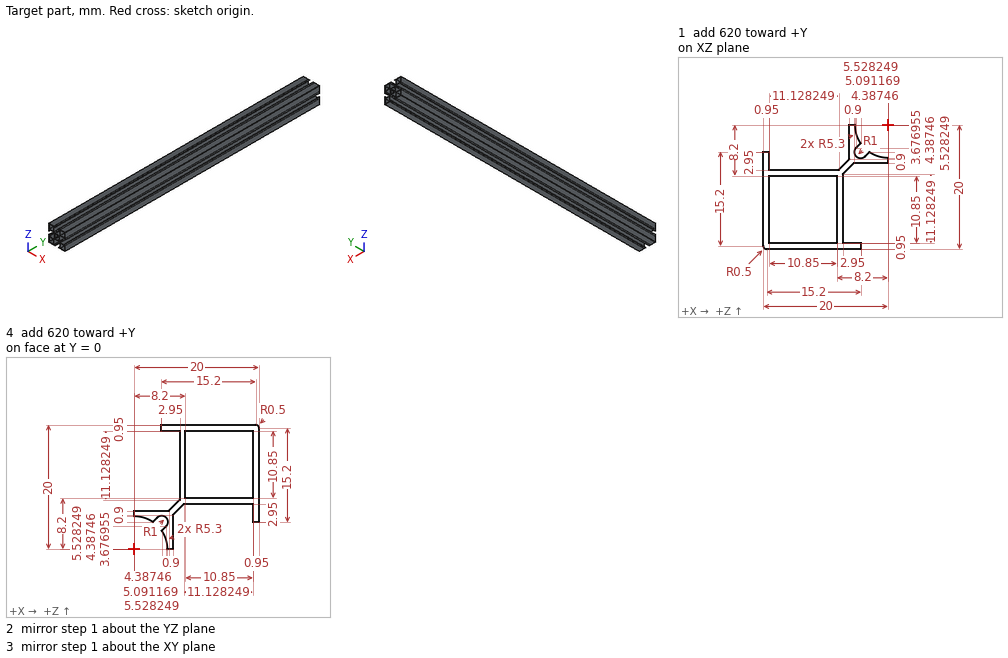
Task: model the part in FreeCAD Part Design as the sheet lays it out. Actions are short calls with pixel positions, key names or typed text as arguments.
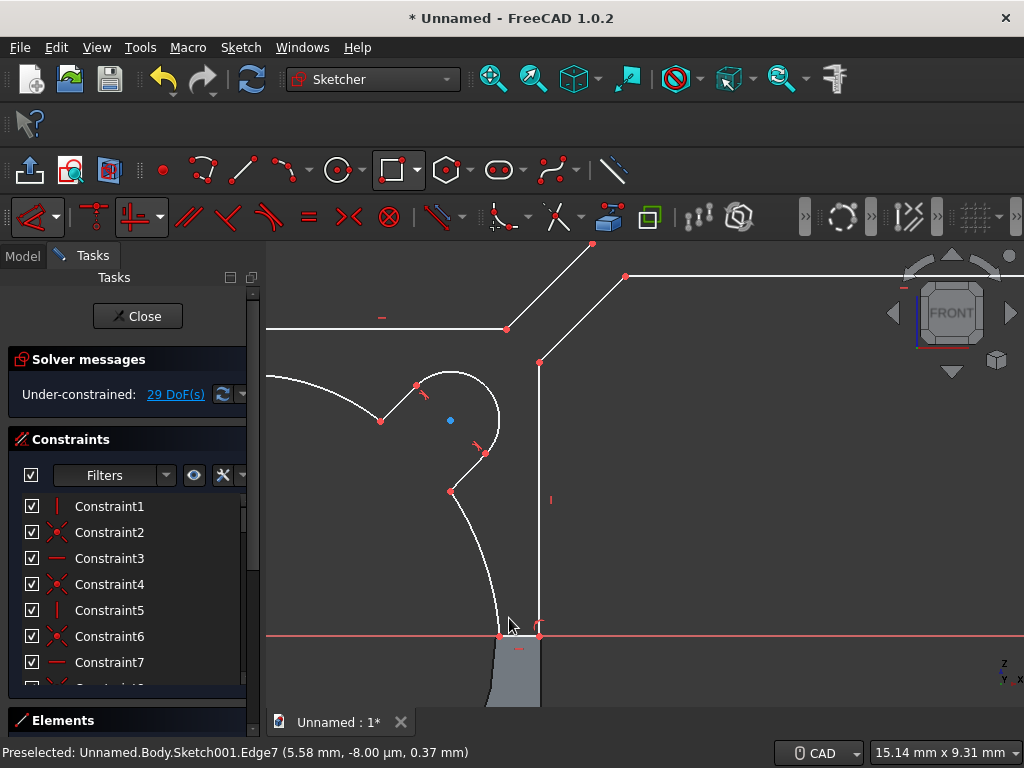
scroll(510, 620, down, 6)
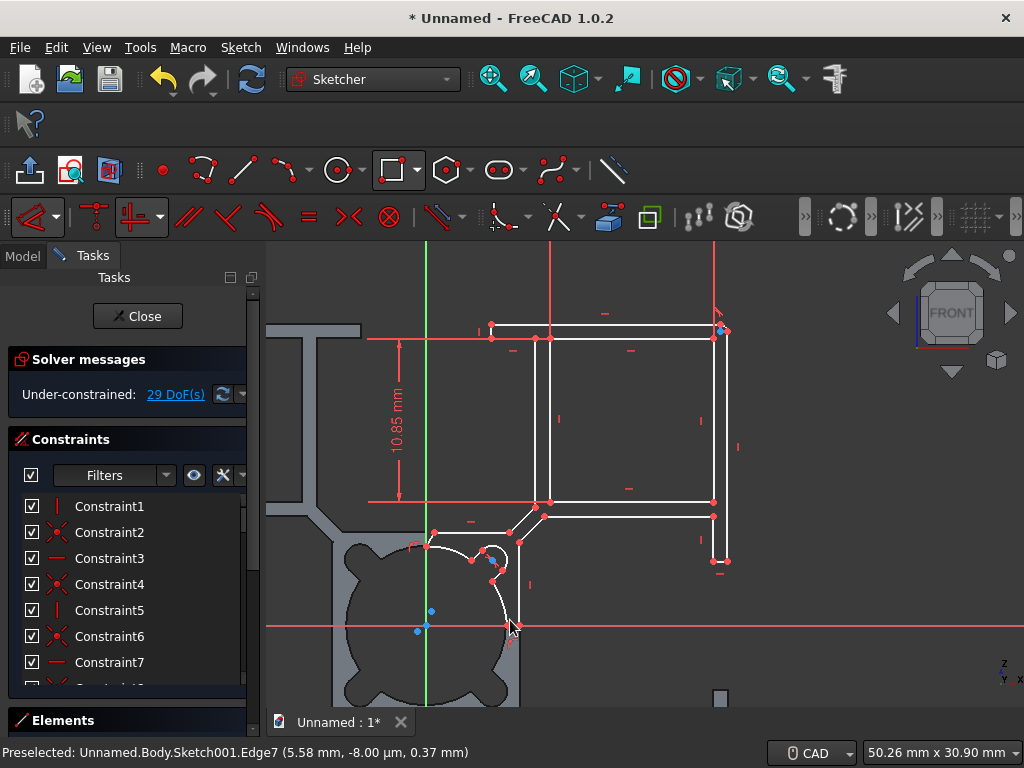
scroll(432, 537, up, 6)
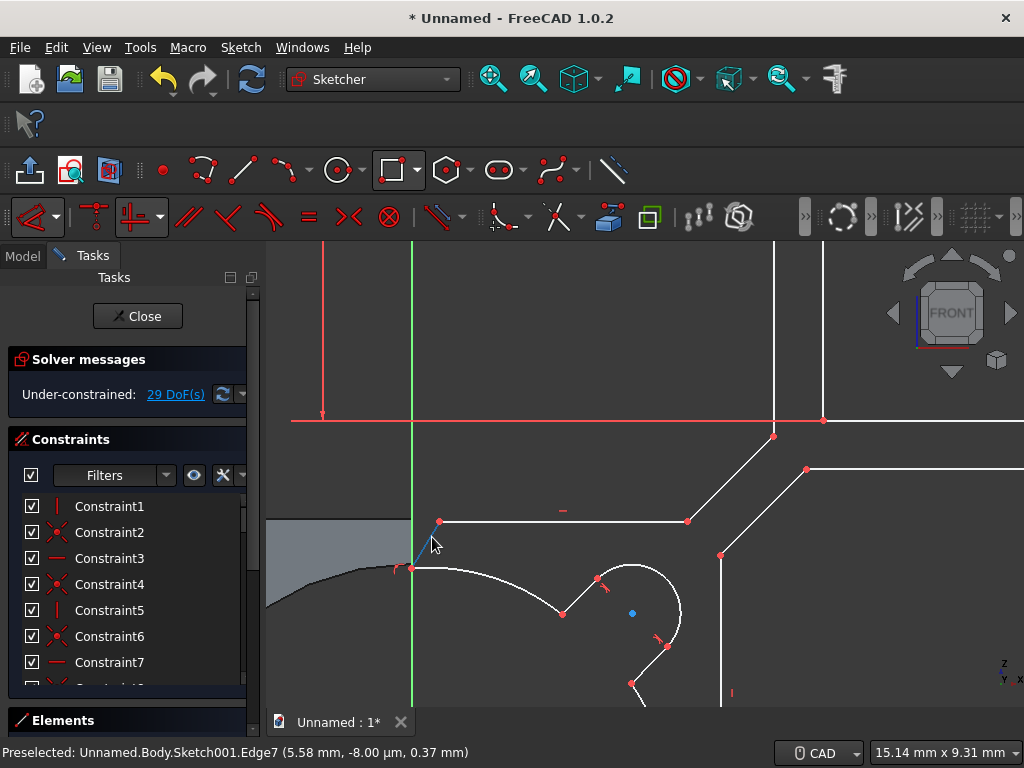
click(431, 536)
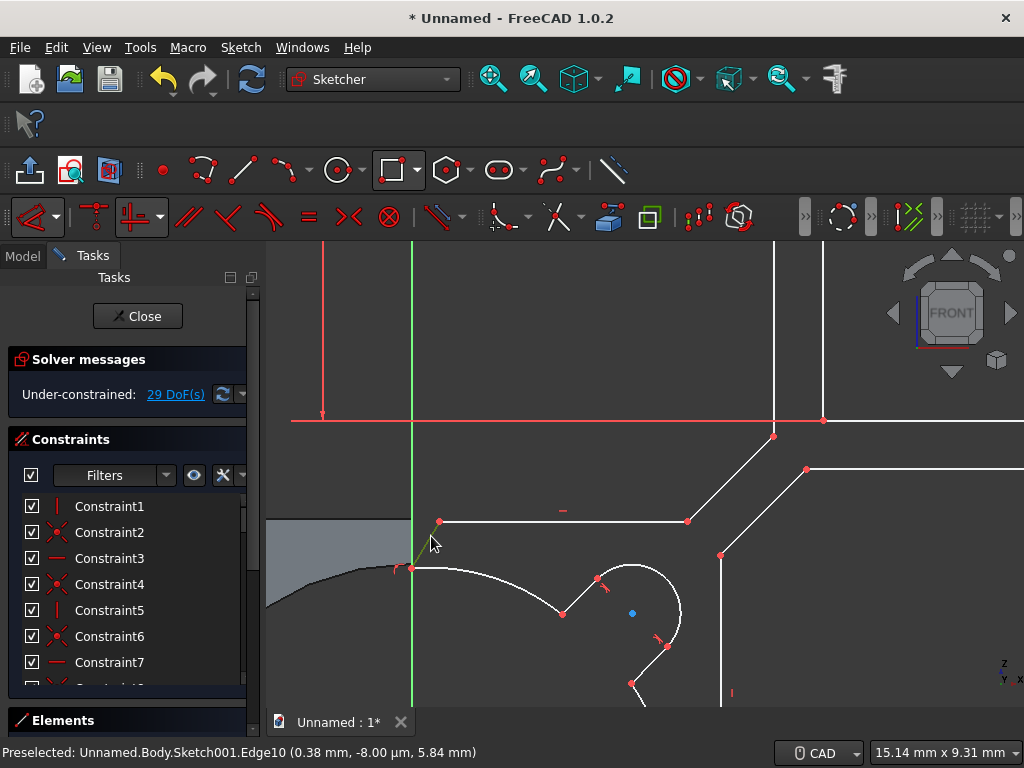
click(162, 218)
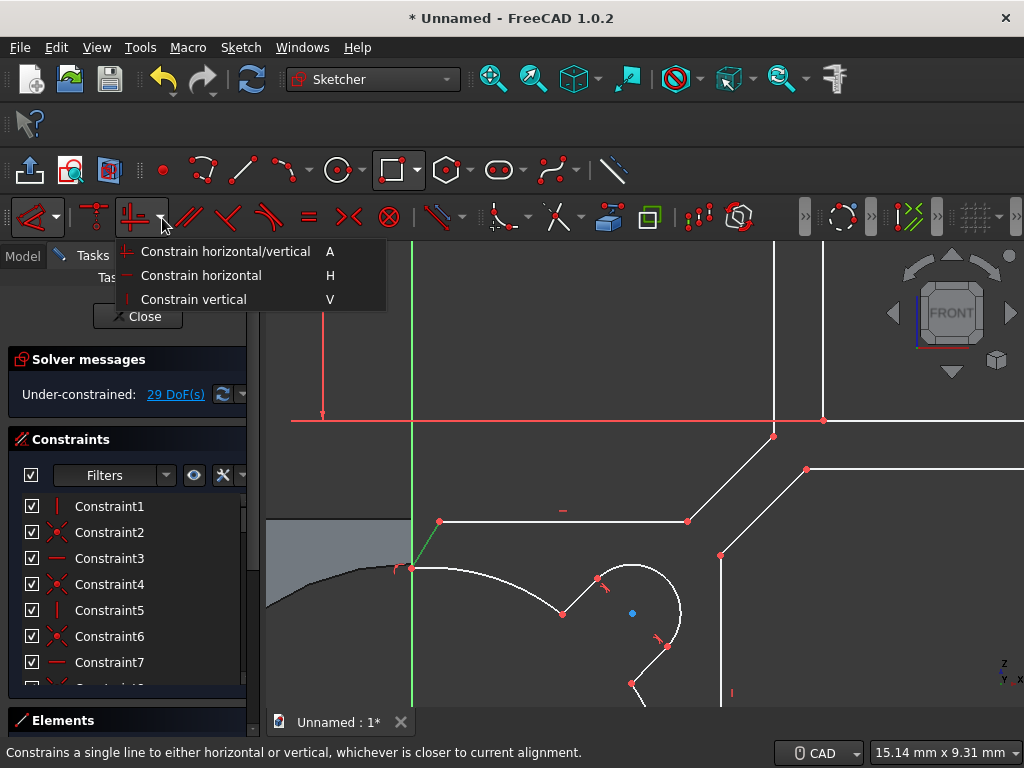
click(251, 299)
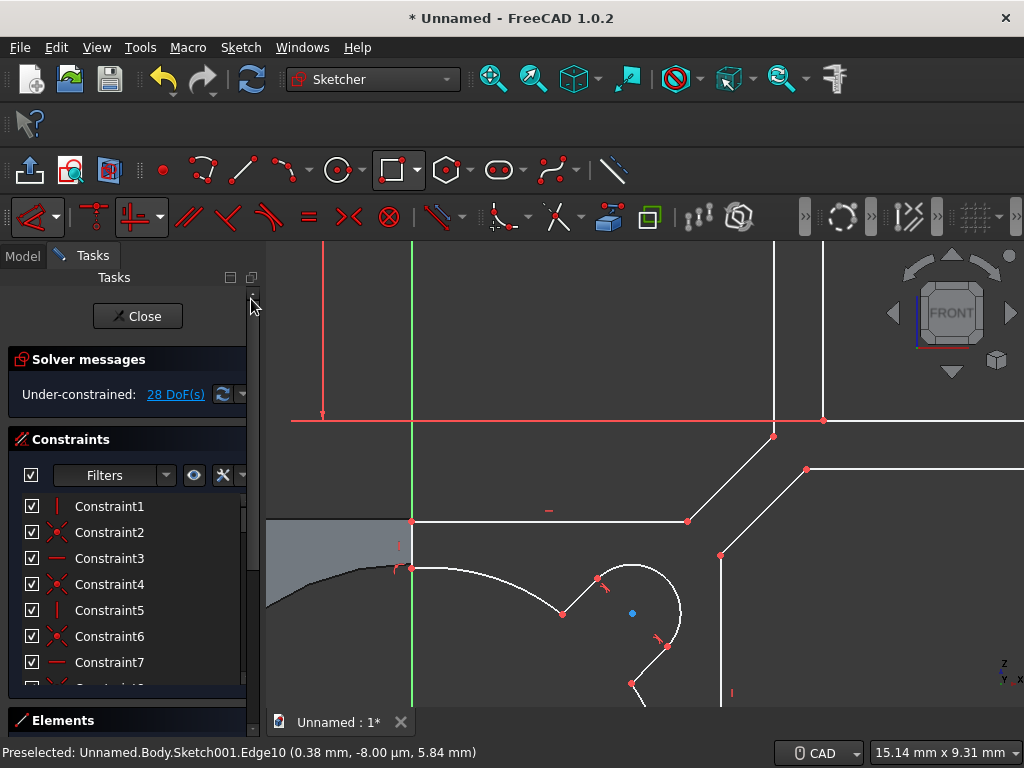
scroll(432, 537, down, 6)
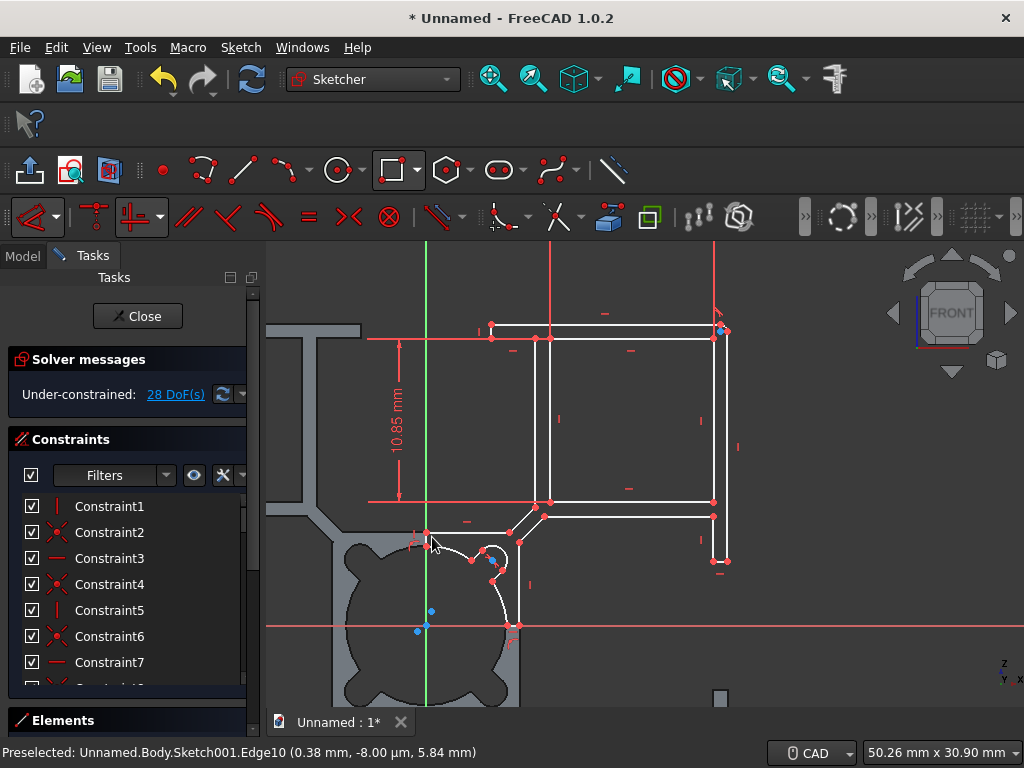
click(505, 612)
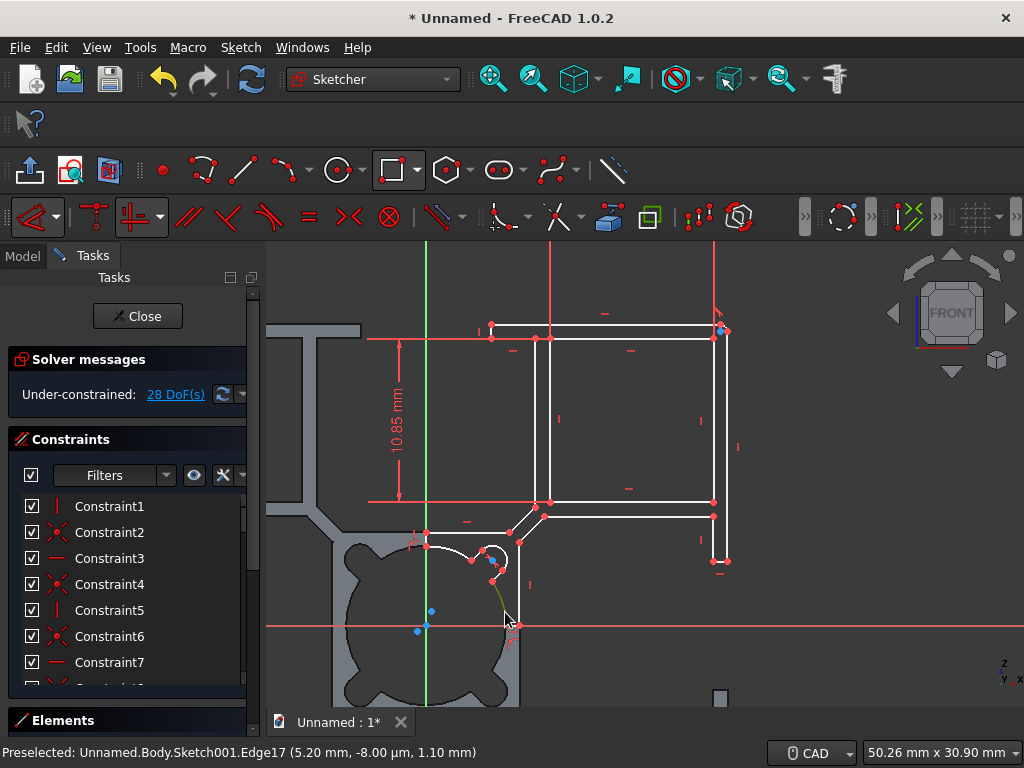
click(459, 553)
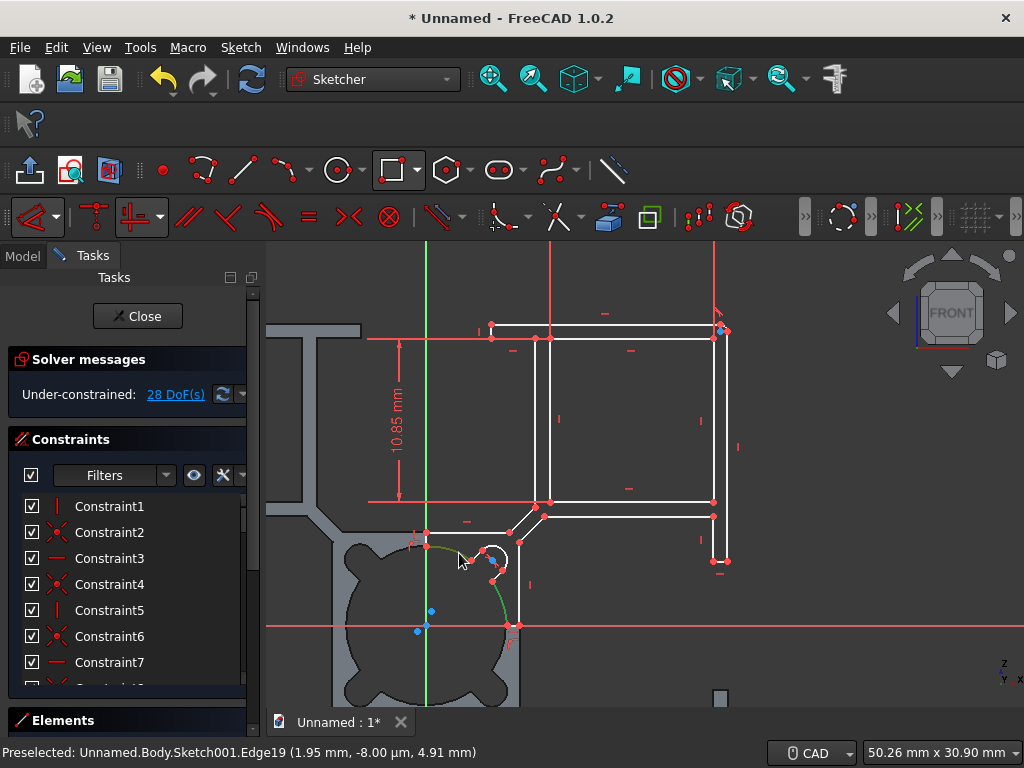
click(94, 218)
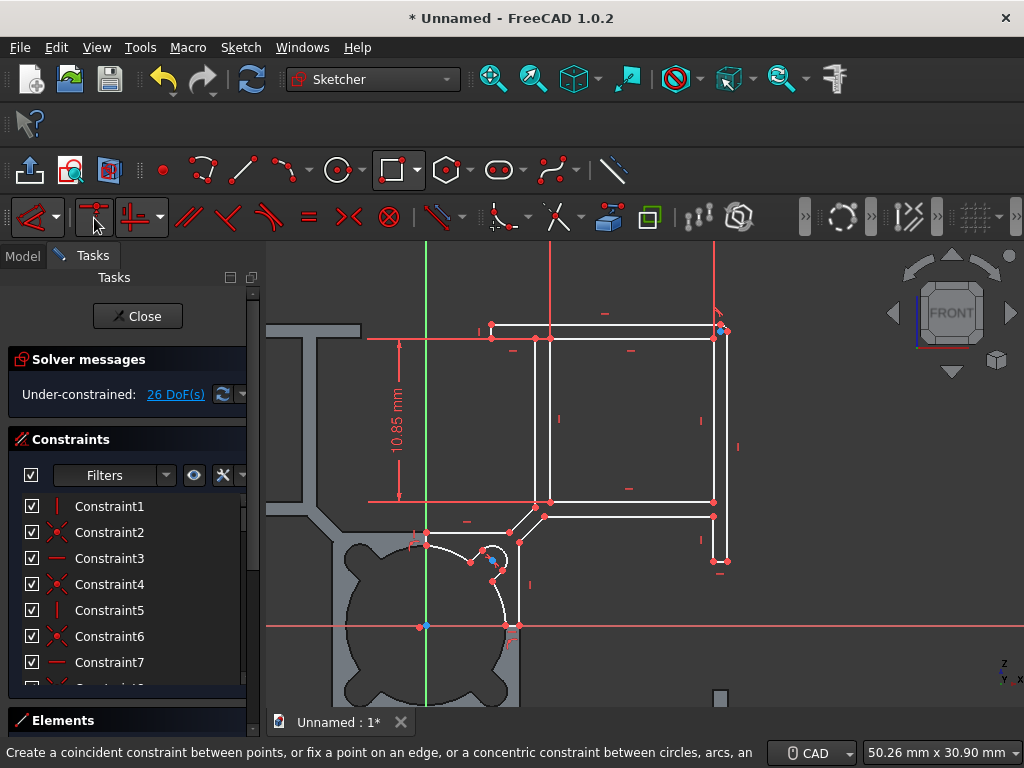
scroll(423, 627, up, 9)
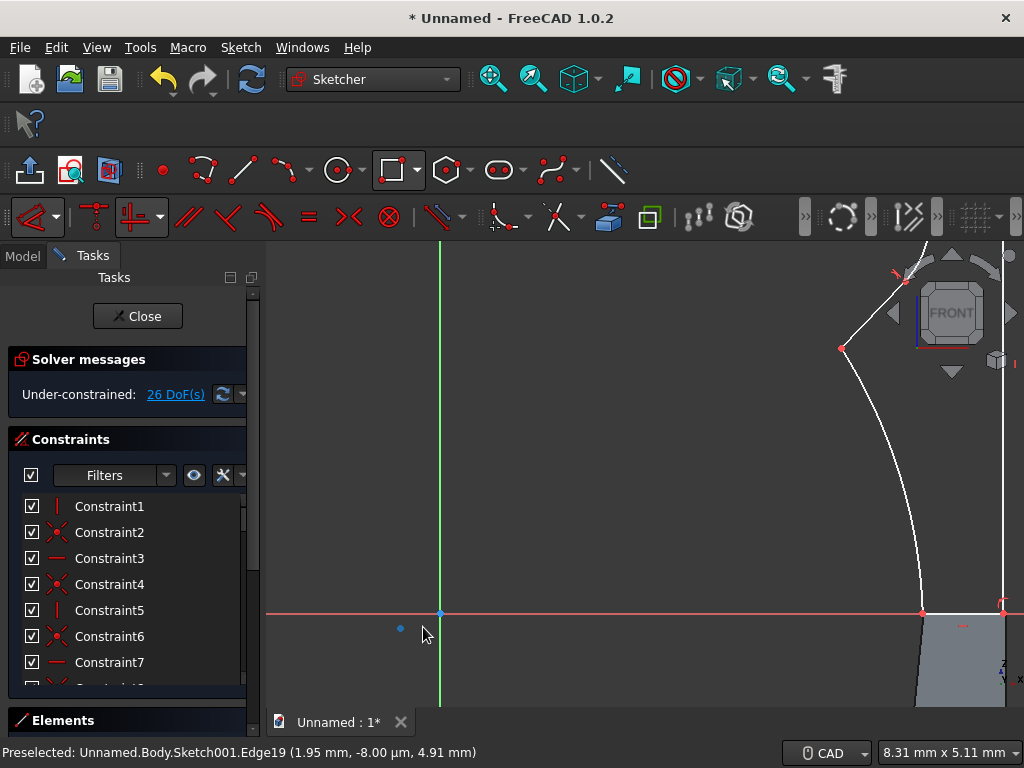
drag(391, 604, 450, 639)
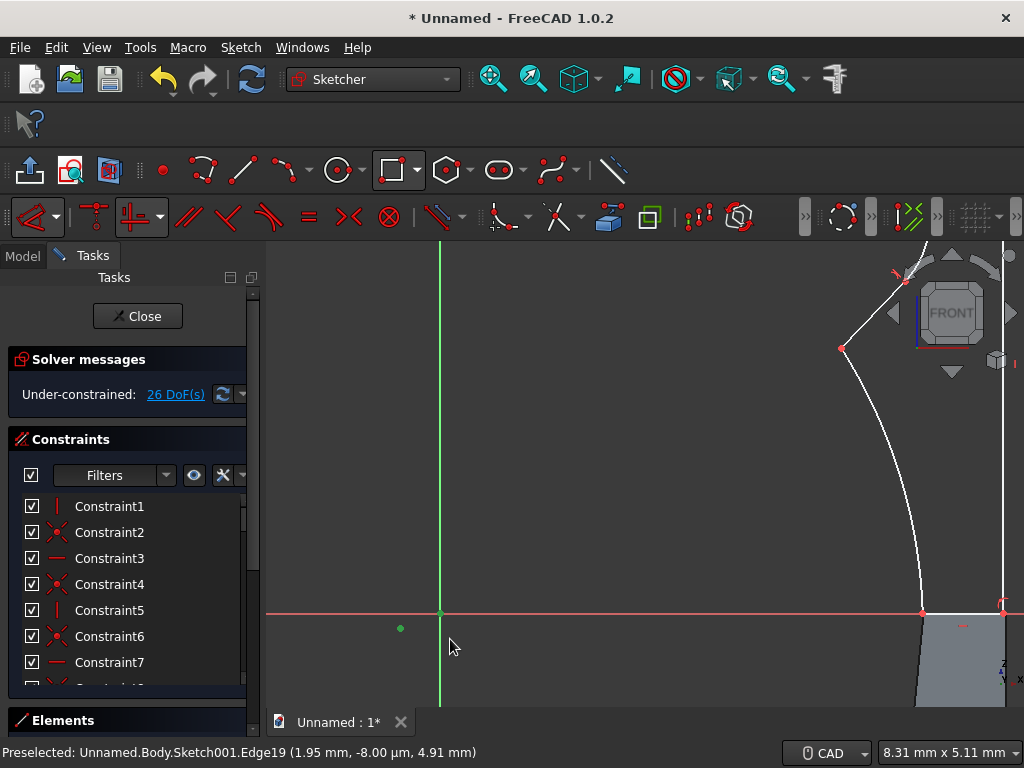
click(94, 218)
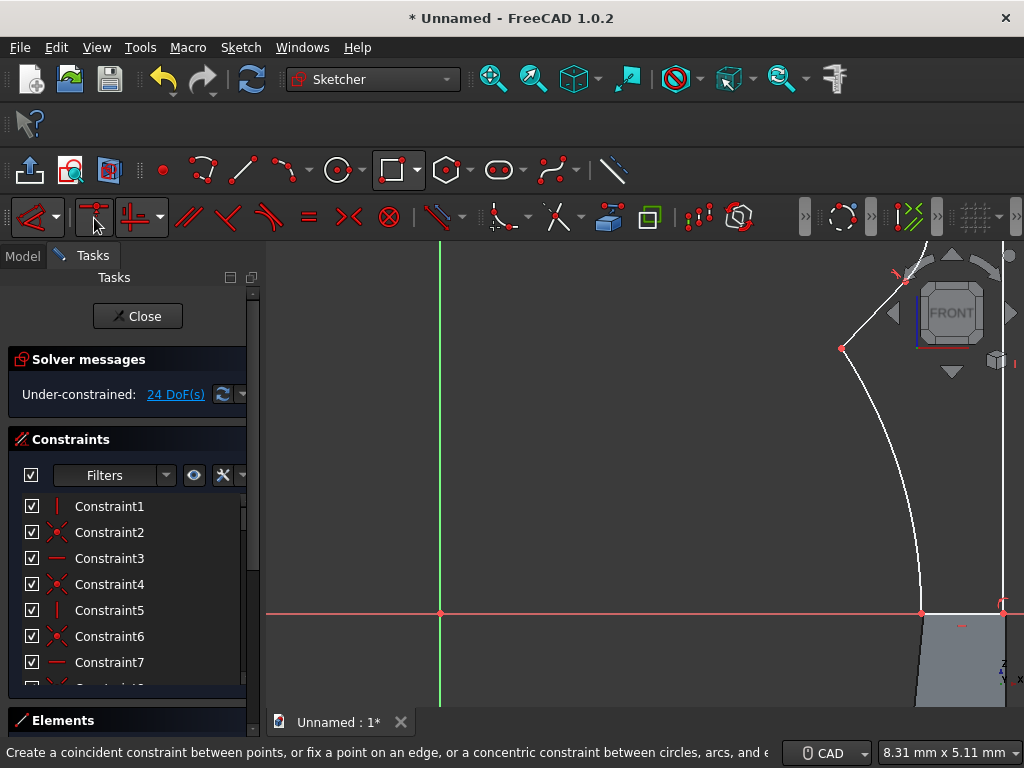
scroll(423, 627, down, 9)